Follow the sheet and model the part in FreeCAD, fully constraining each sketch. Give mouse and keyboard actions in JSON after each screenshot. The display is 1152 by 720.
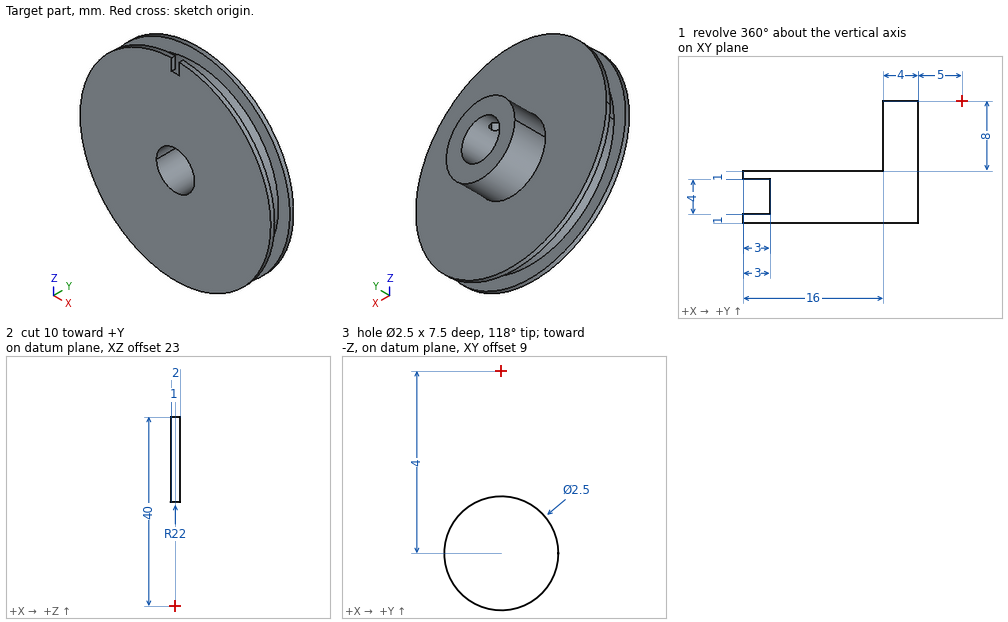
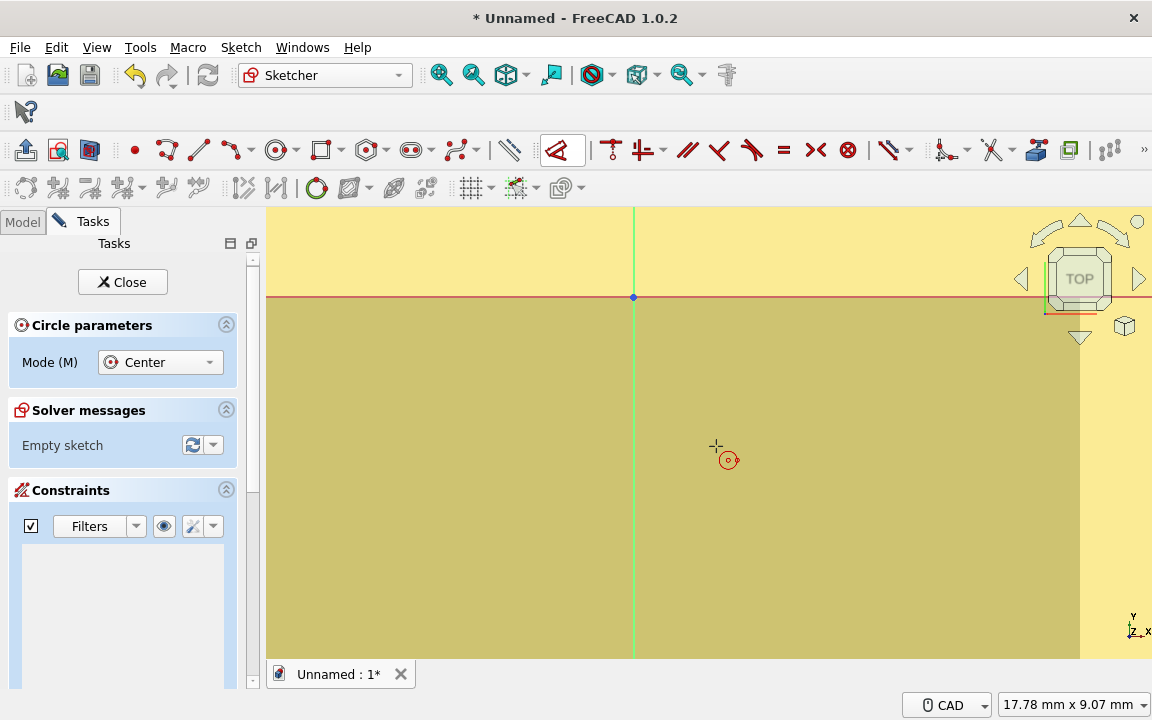
{"action": "left_click", "coordinate": [634, 497]}
{"action": "left_click", "coordinate": [678, 453]}
{"action": "key", "text": "Escape"}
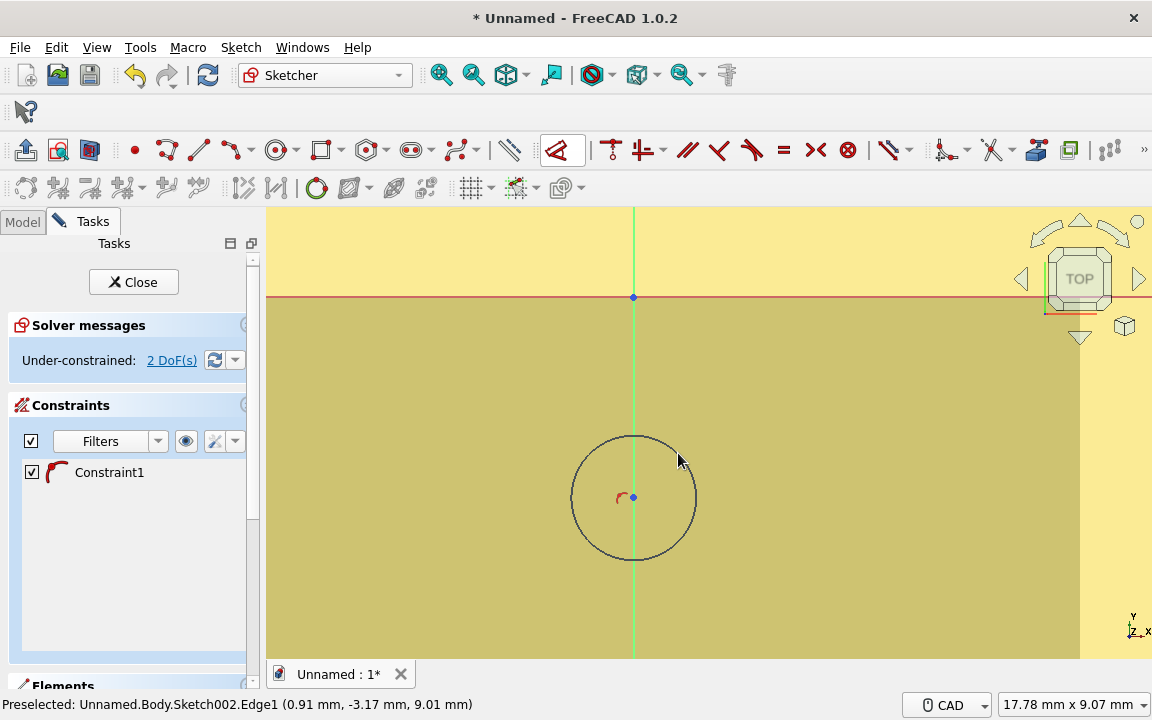
{"action": "left_click", "coordinate": [678, 454]}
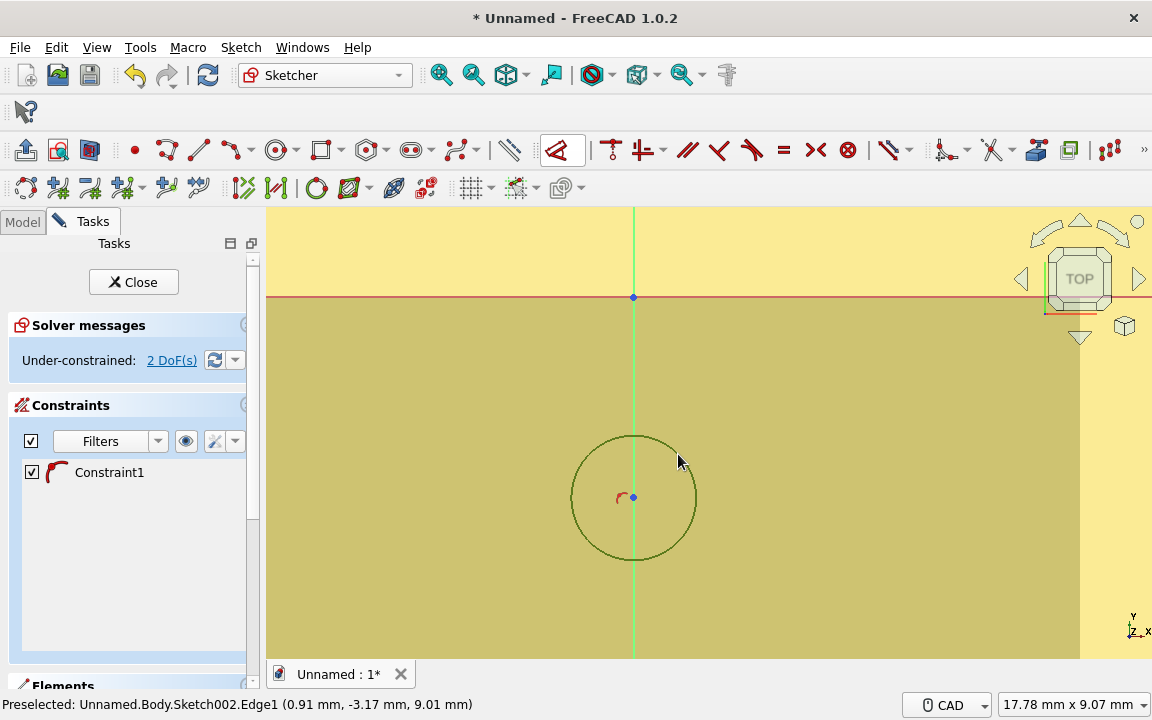
{"action": "key", "text": "k o"}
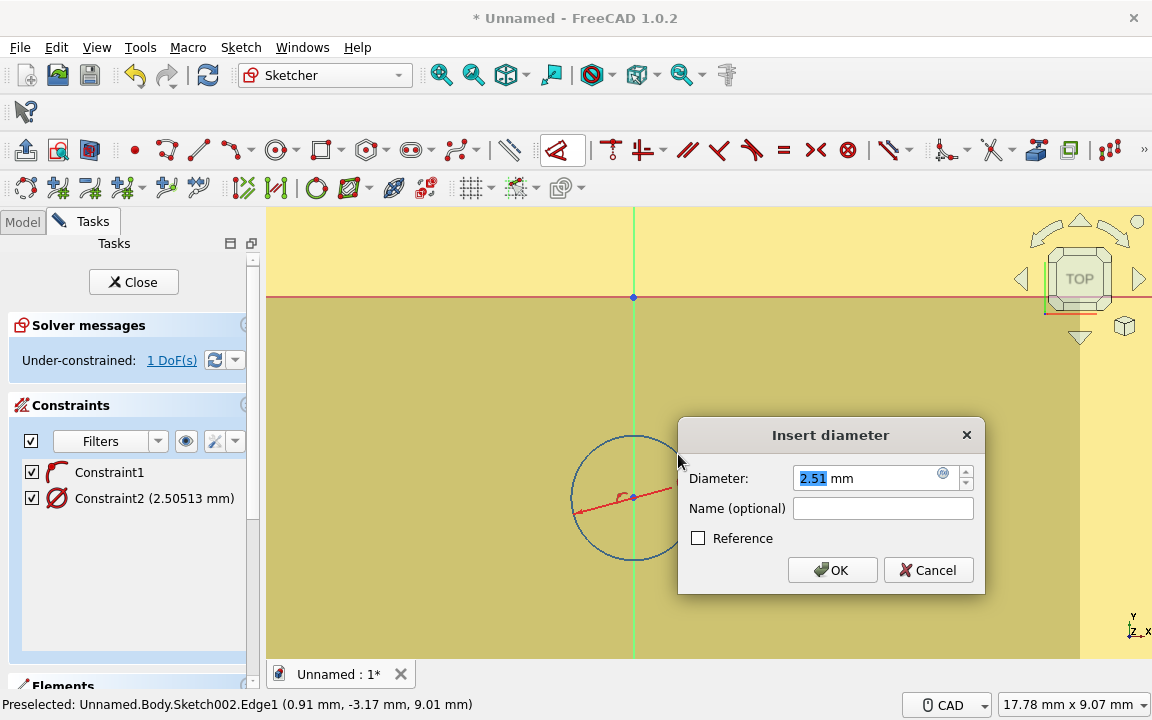
{"action": "type", "text": "2.5"}
{"action": "key", "text": "Return"}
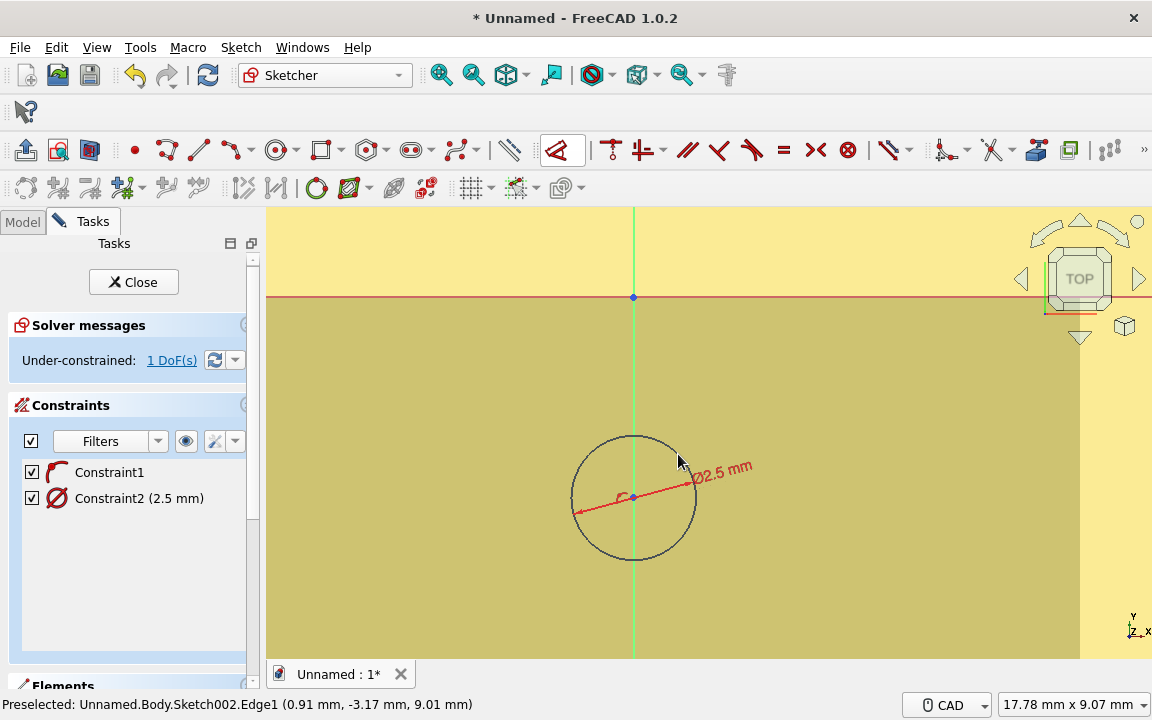
{"action": "left_click", "coordinate": [634, 498]}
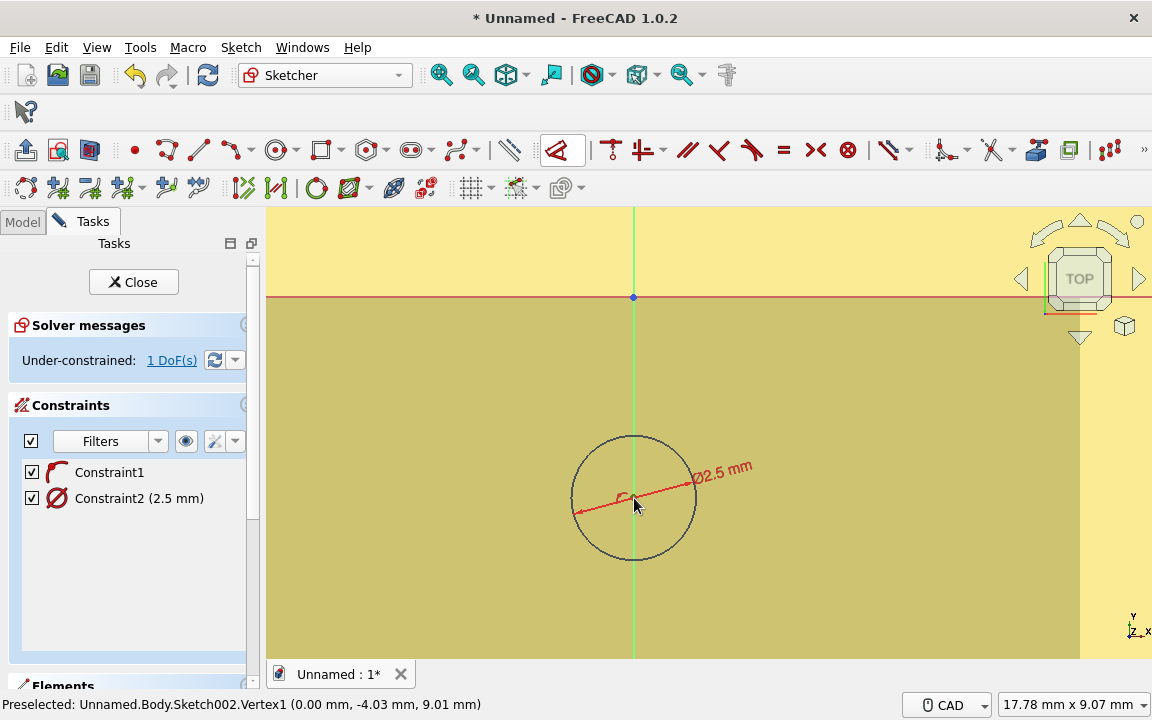
{"action": "key", "text": "i"}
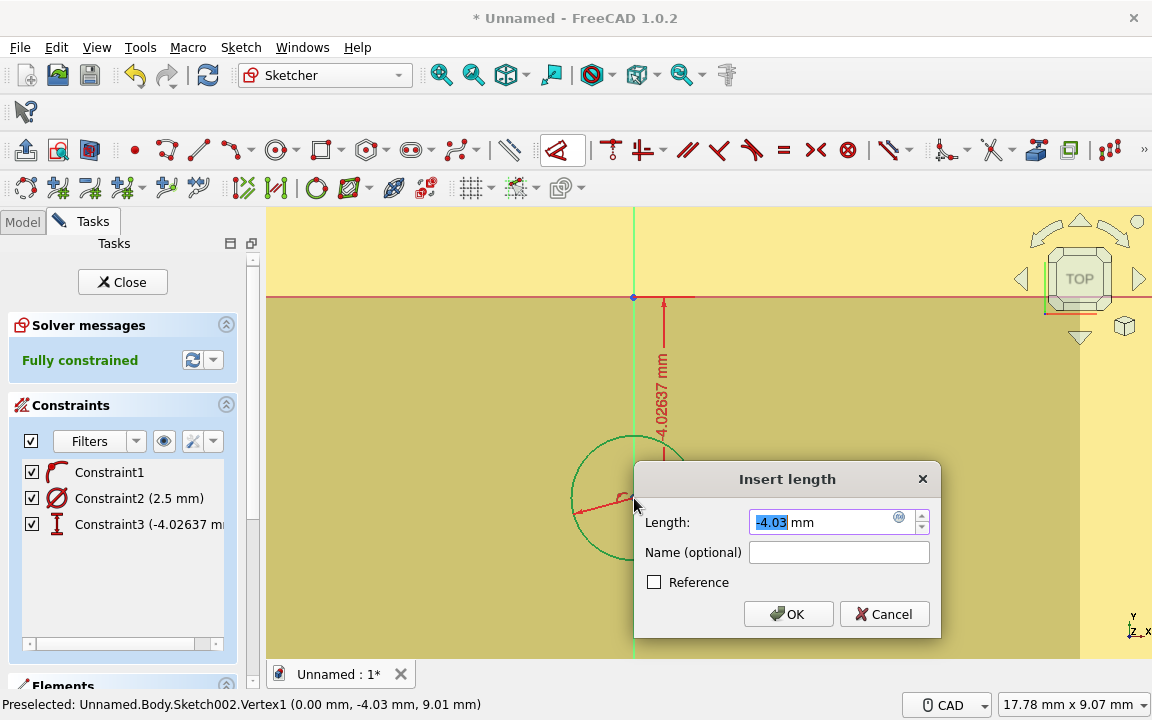
{"action": "type", "text": "-4"}
{"action": "key", "text": "Return"}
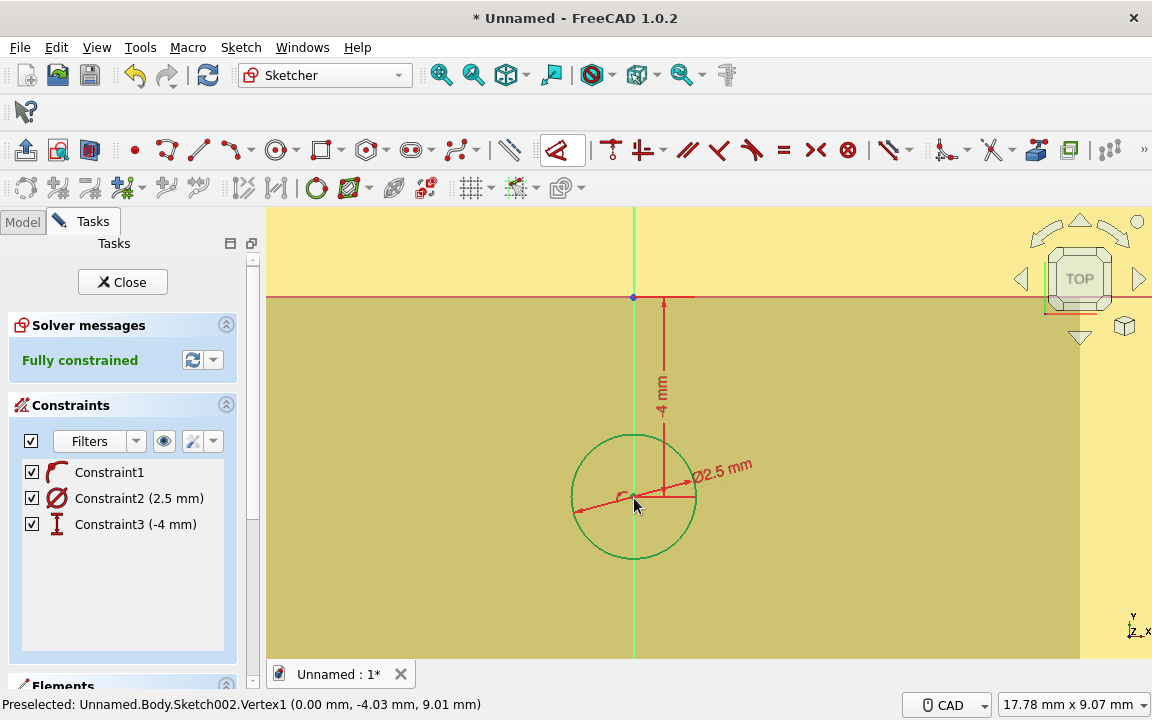
{"action": "left_click", "coordinate": [123, 282]}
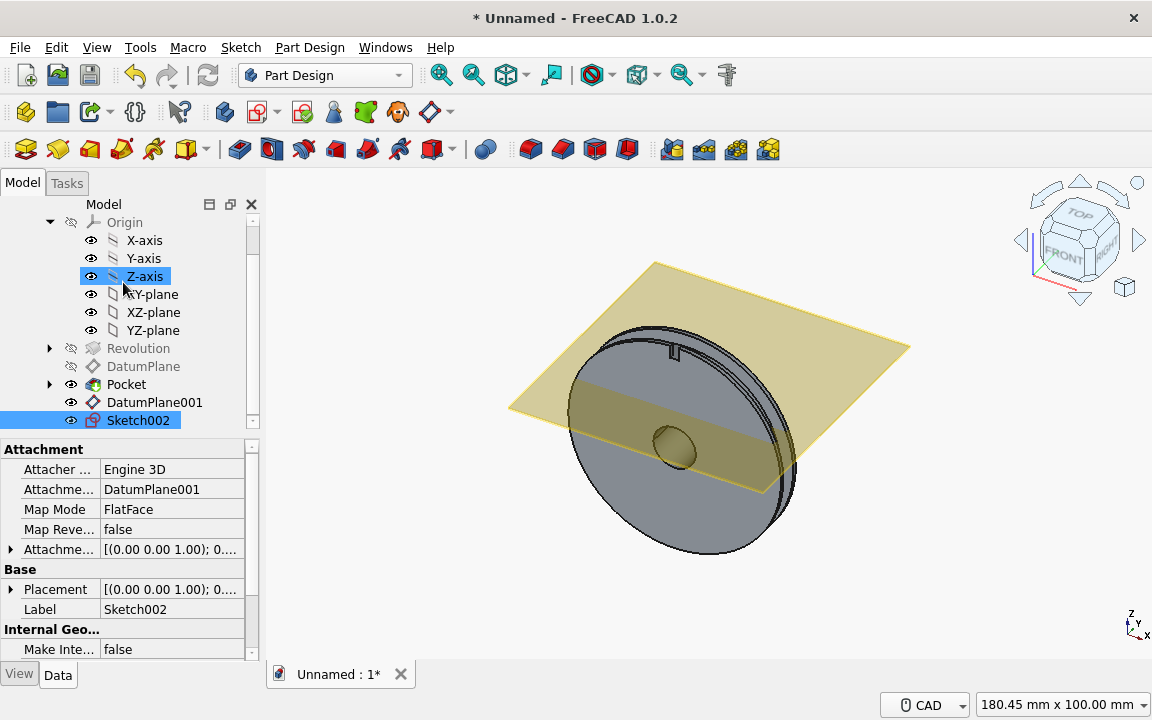
{"action": "left_click", "coordinate": [272, 150]}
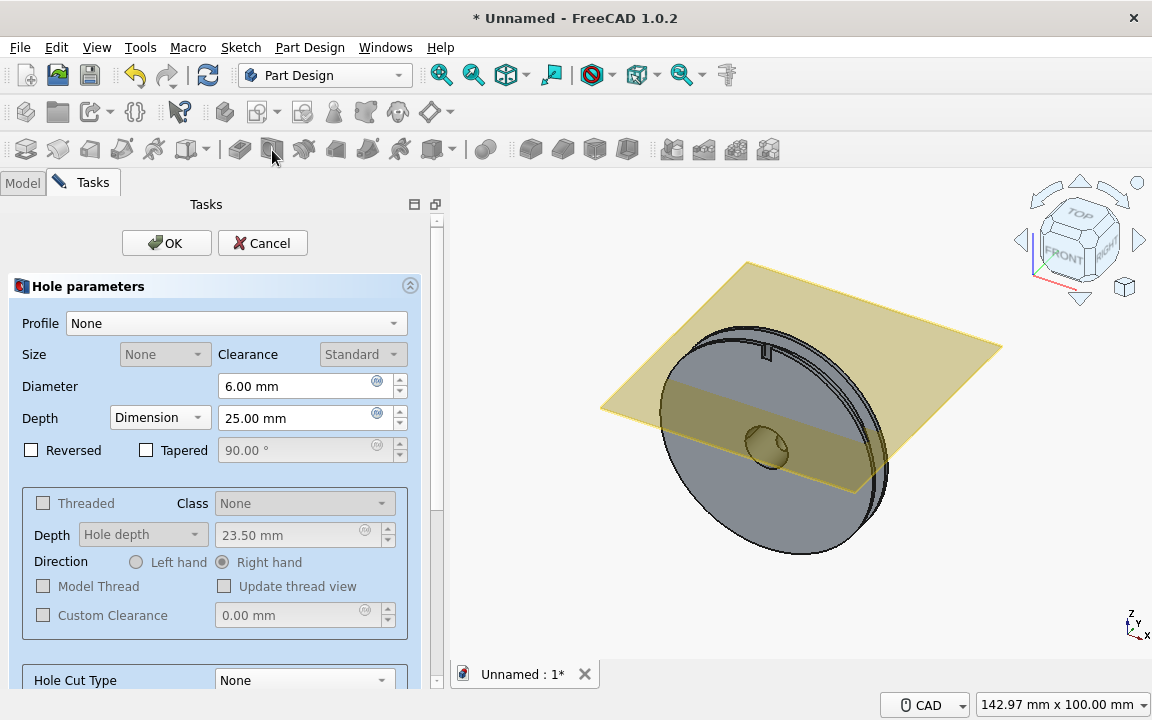
{"action": "triple_click", "coordinate": [305, 386]}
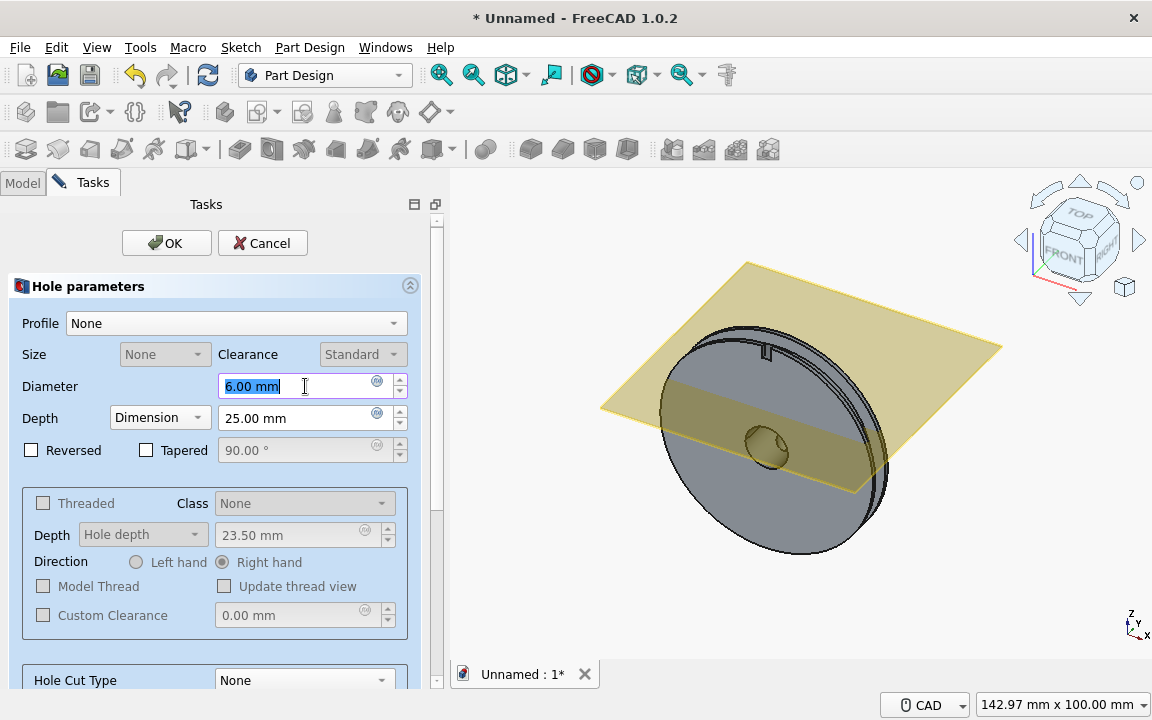
{"action": "type", "text": "2.5"}
{"action": "key", "text": "Tab"}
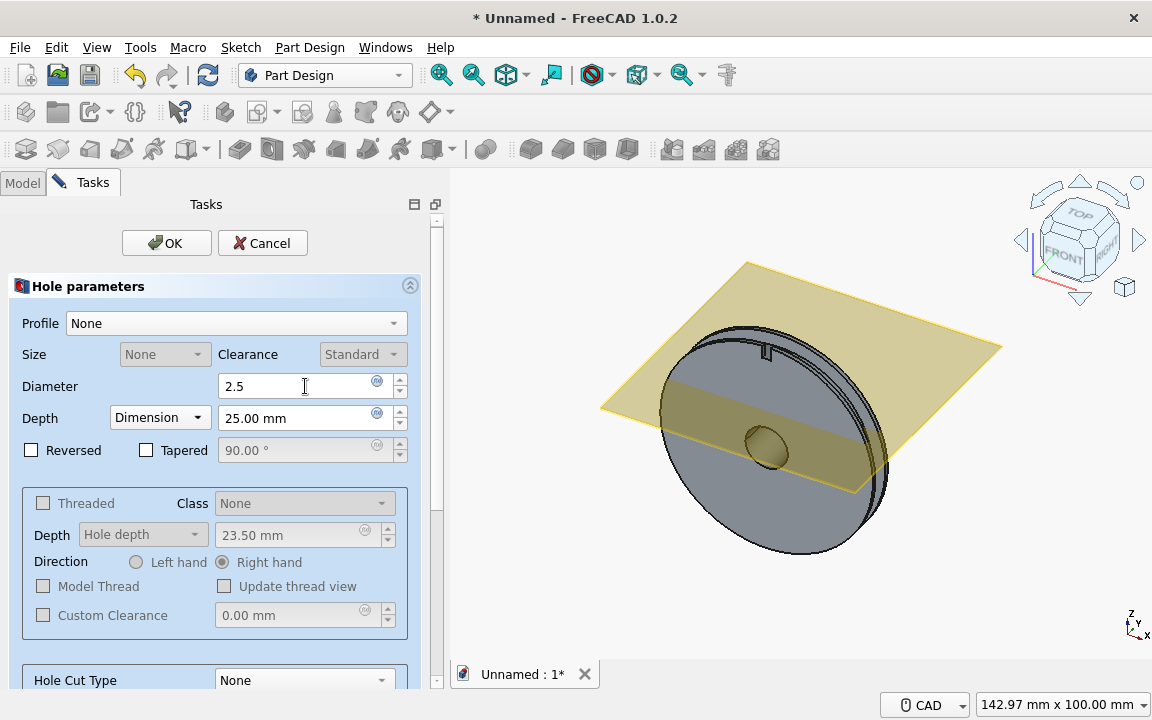
{"action": "triple_click", "coordinate": [305, 418]}